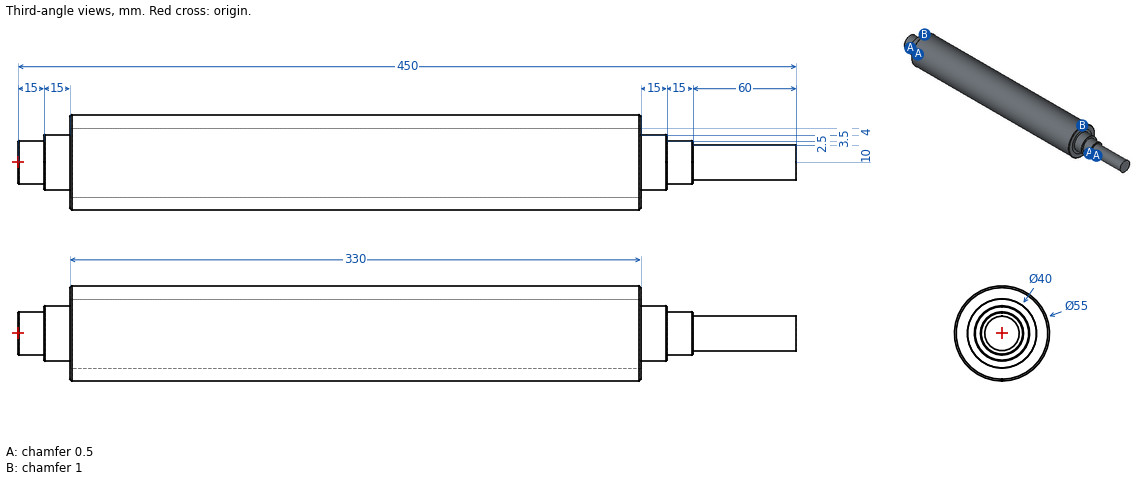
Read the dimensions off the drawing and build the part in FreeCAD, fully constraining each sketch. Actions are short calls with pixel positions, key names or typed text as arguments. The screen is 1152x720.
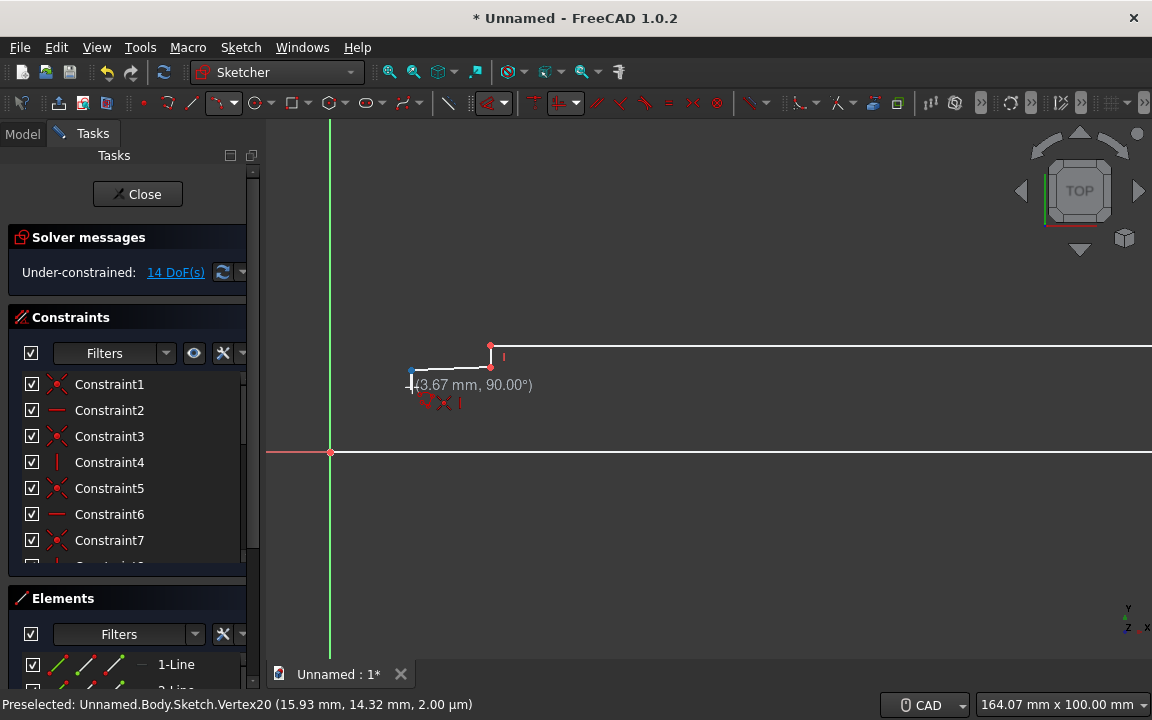
click(411, 385)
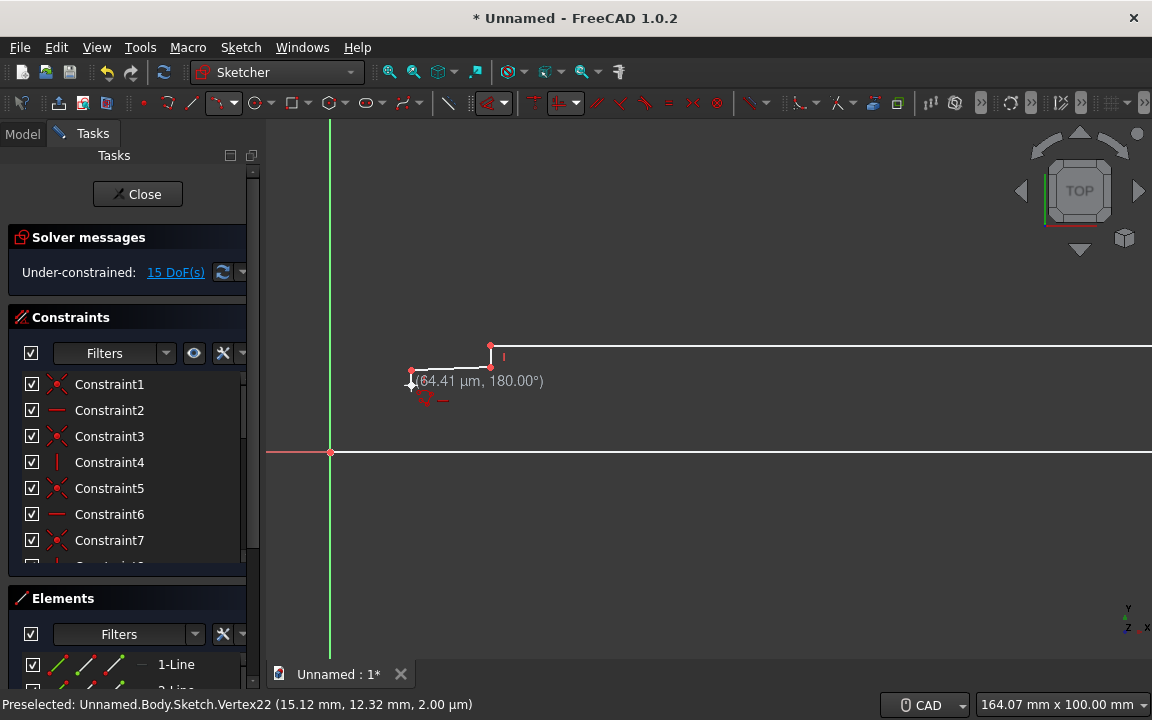
scroll(412, 387, down, 8)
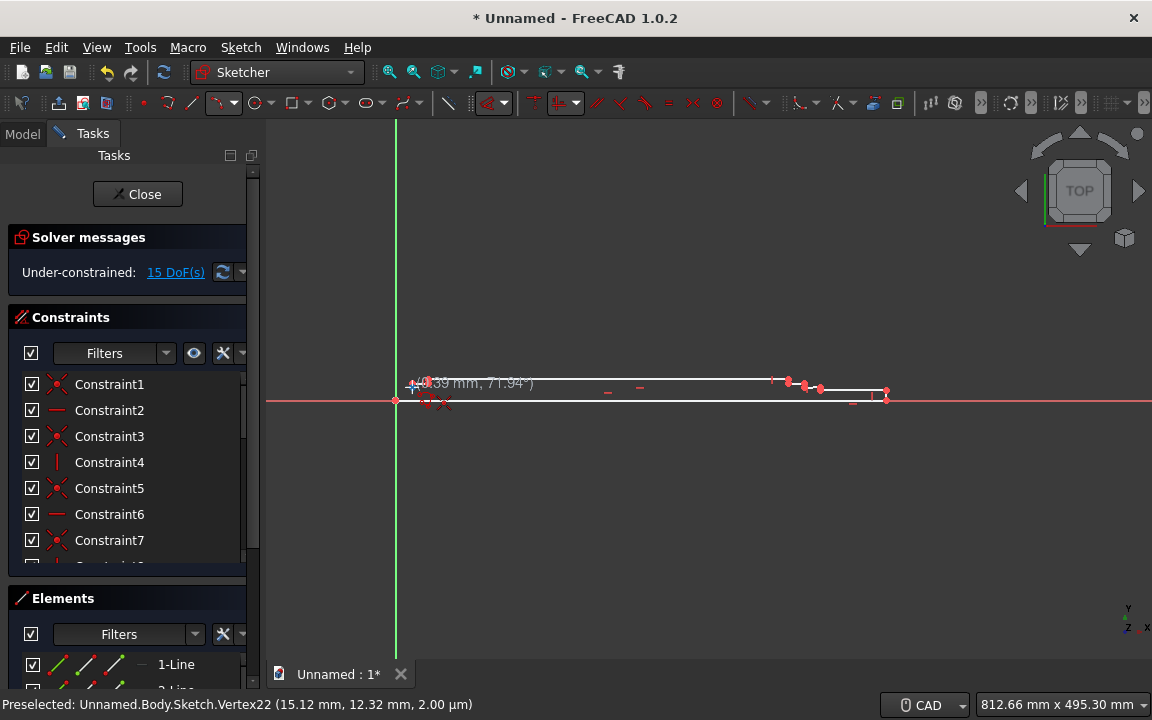
click(405, 387)
click(396, 401)
key(Escape)
key(Escape)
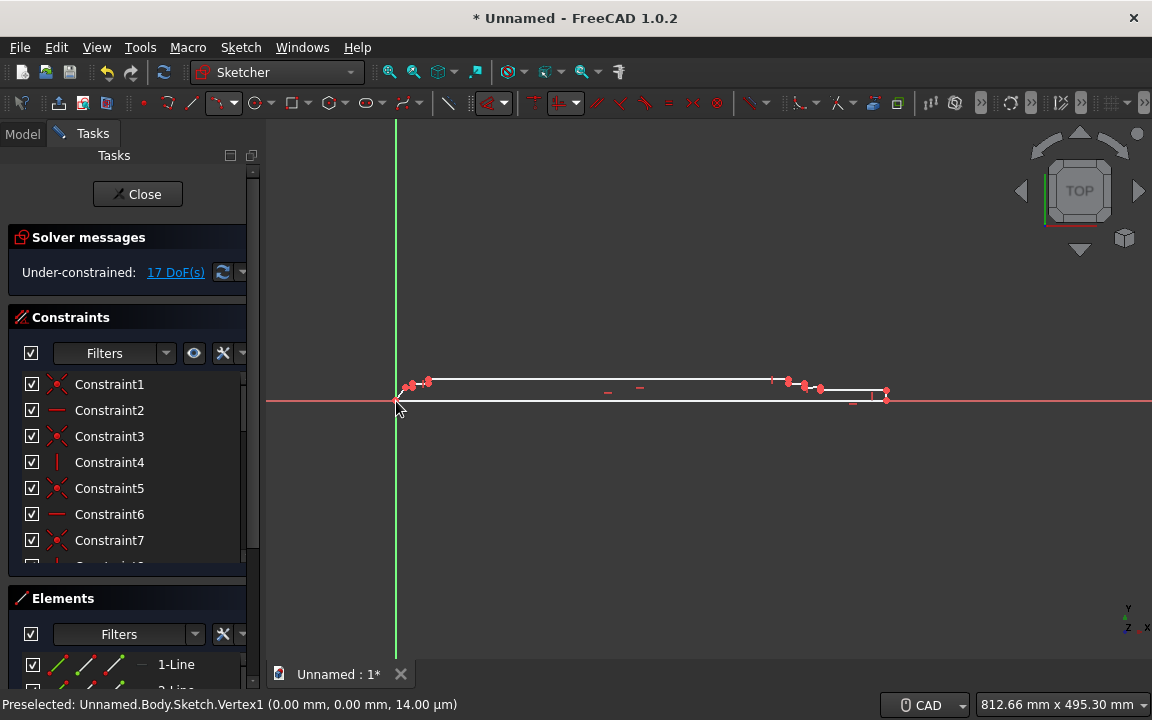
scroll(812, 388, up, 3)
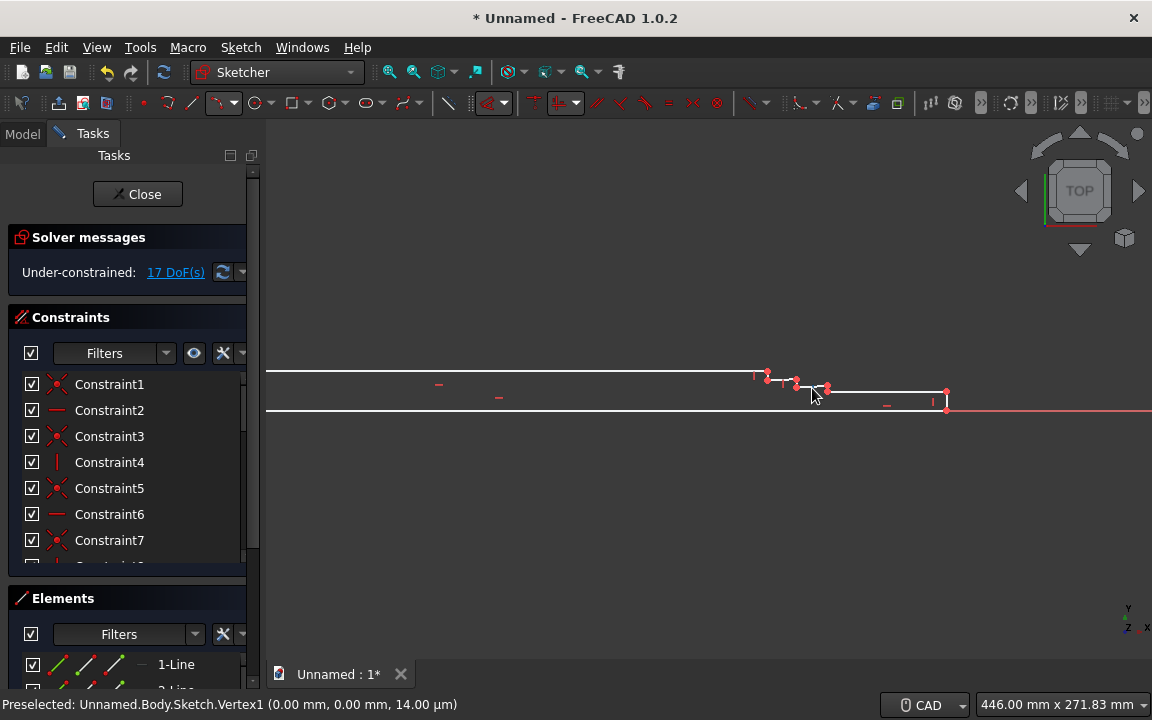
click(806, 387)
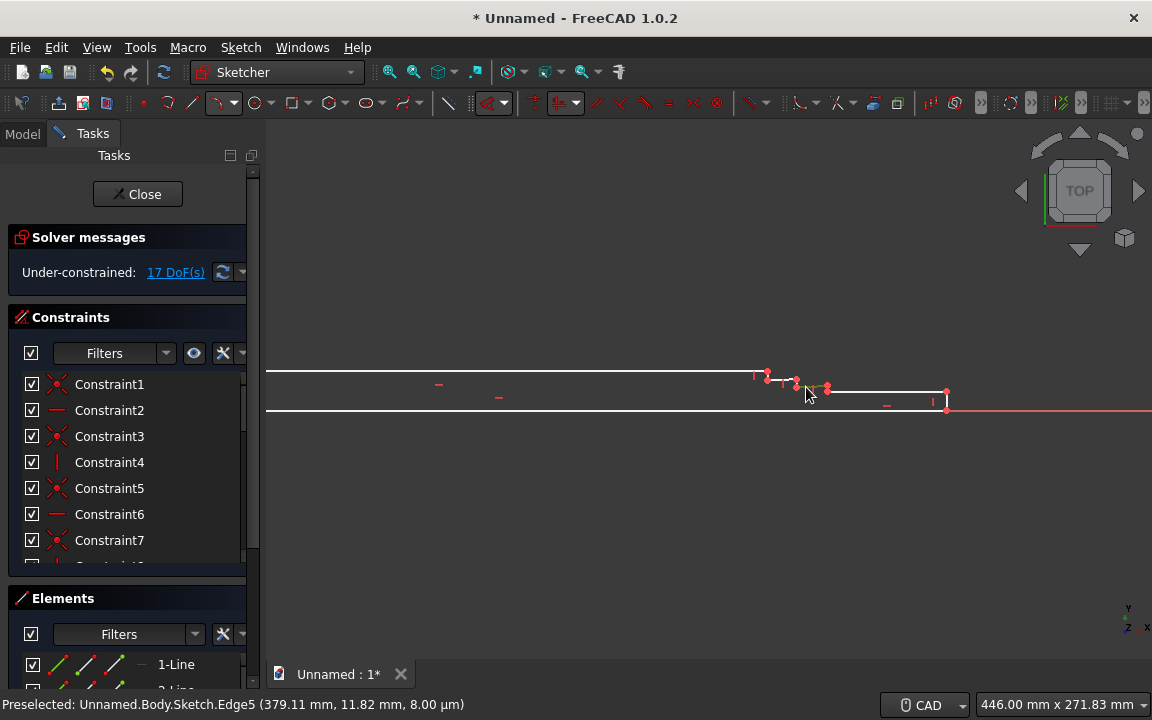
key(h)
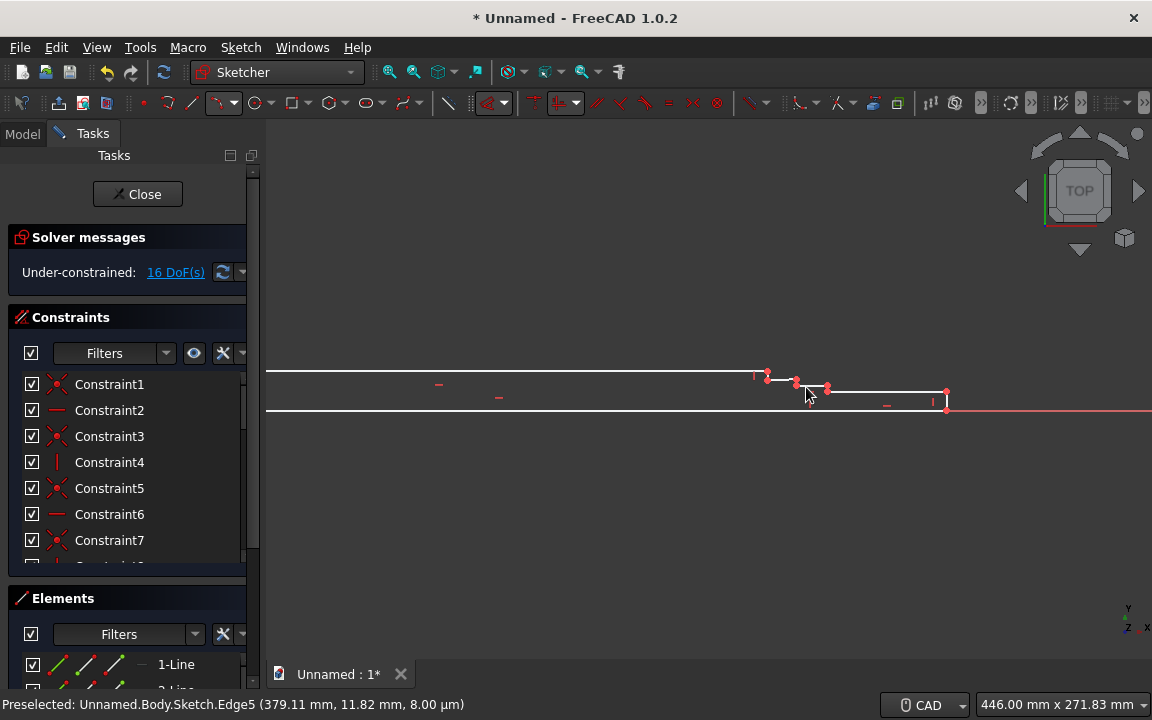
click(785, 380)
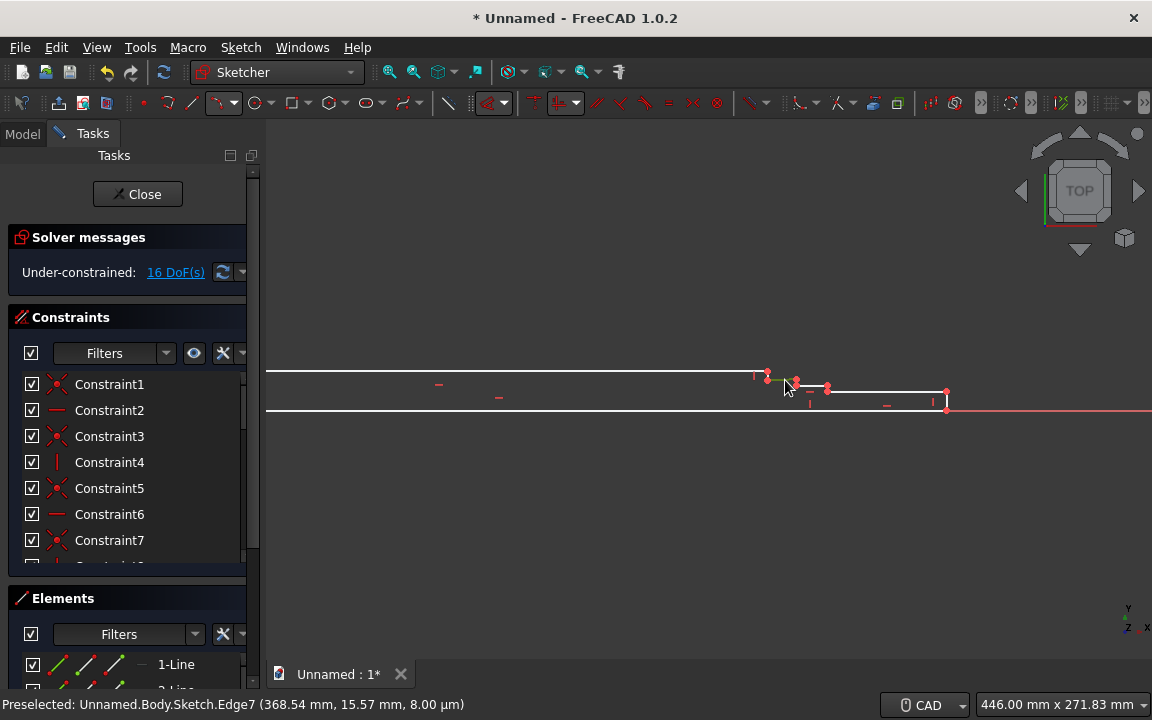
click(578, 104)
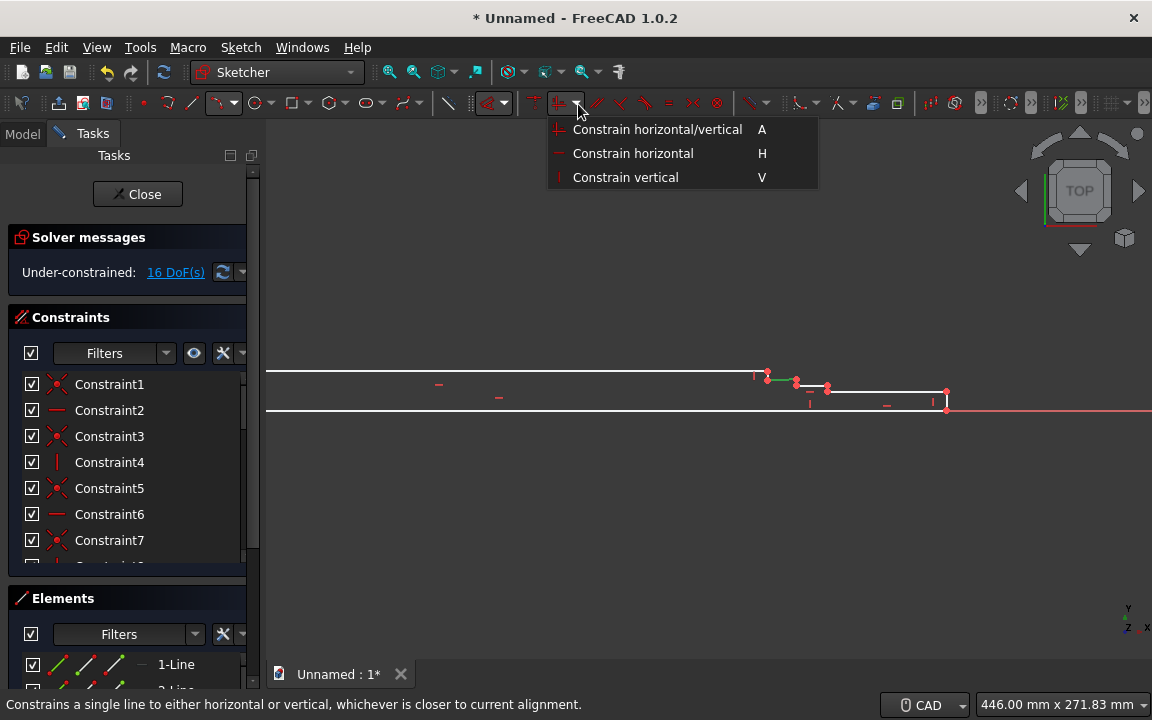
click(683, 153)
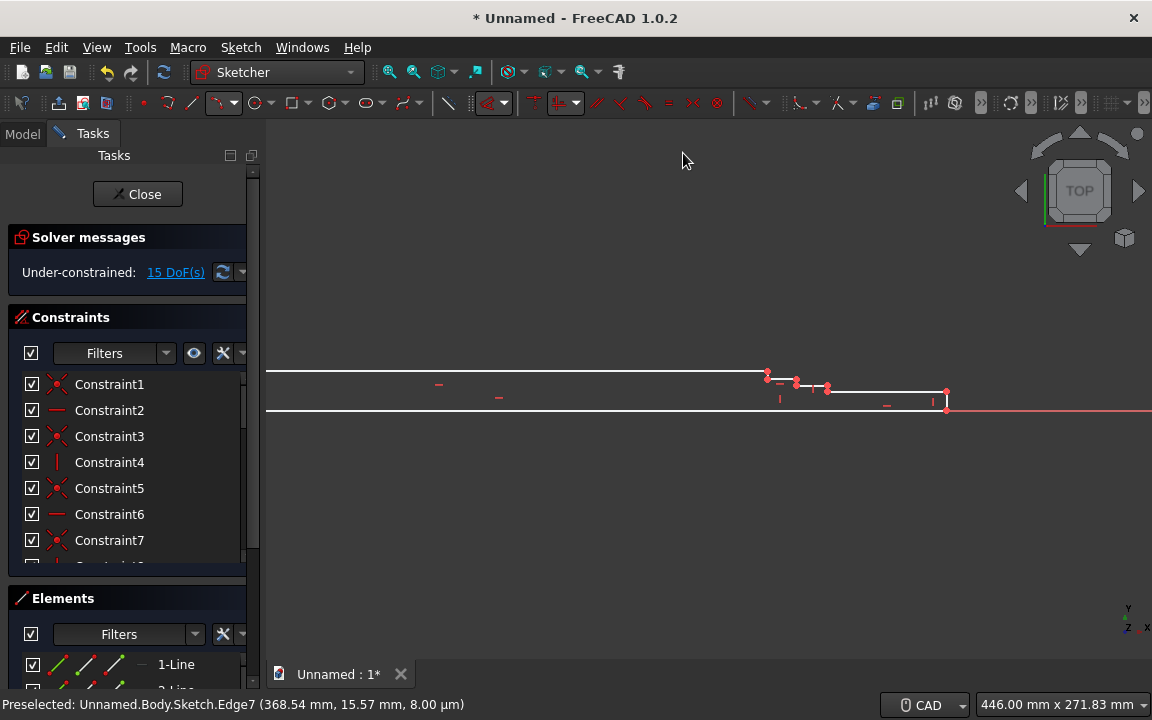
scroll(812, 387, down, 3)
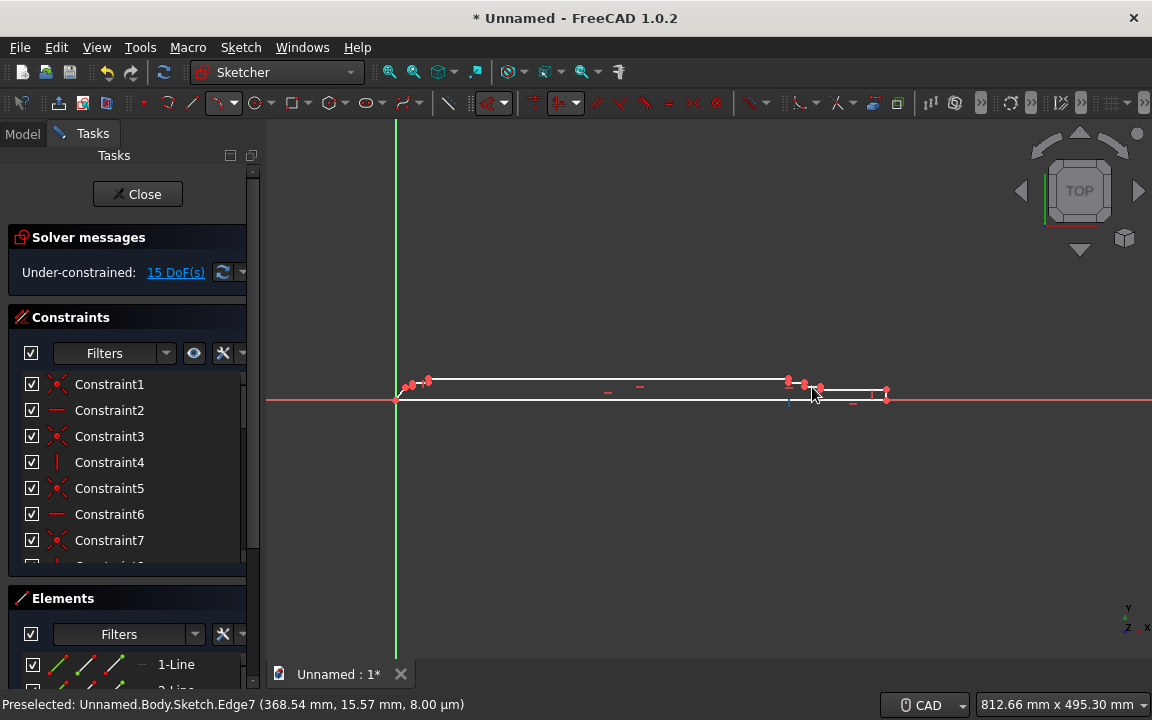
scroll(422, 383, up, 4)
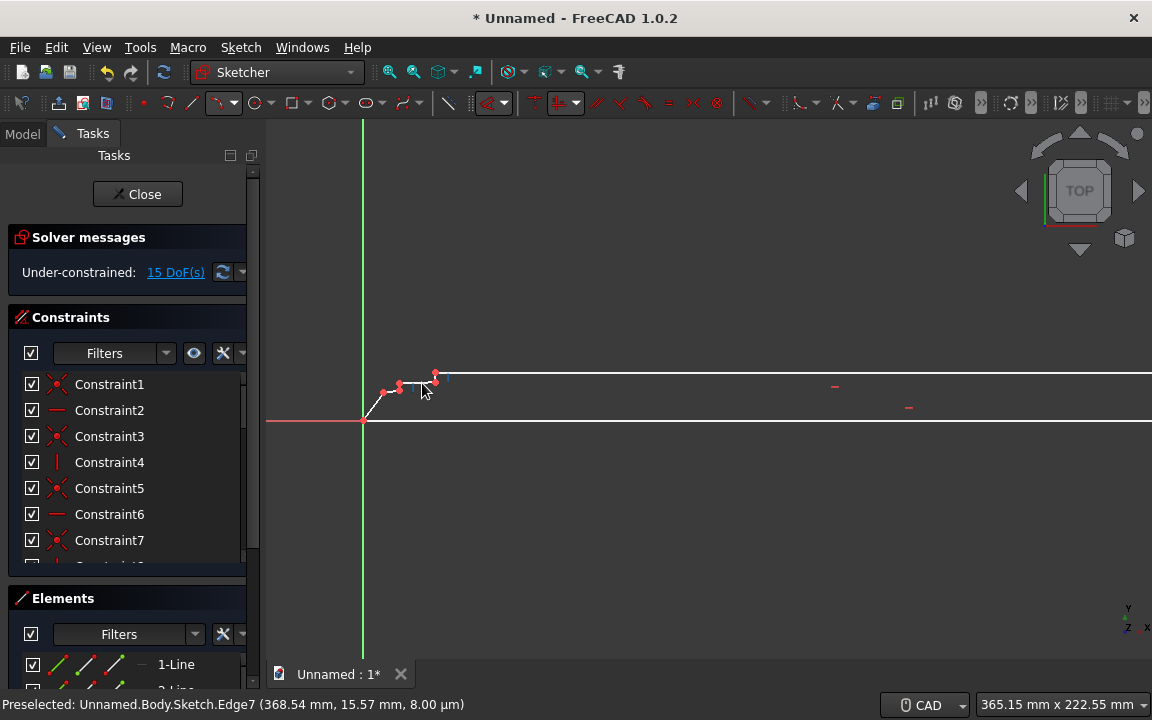
click(421, 383)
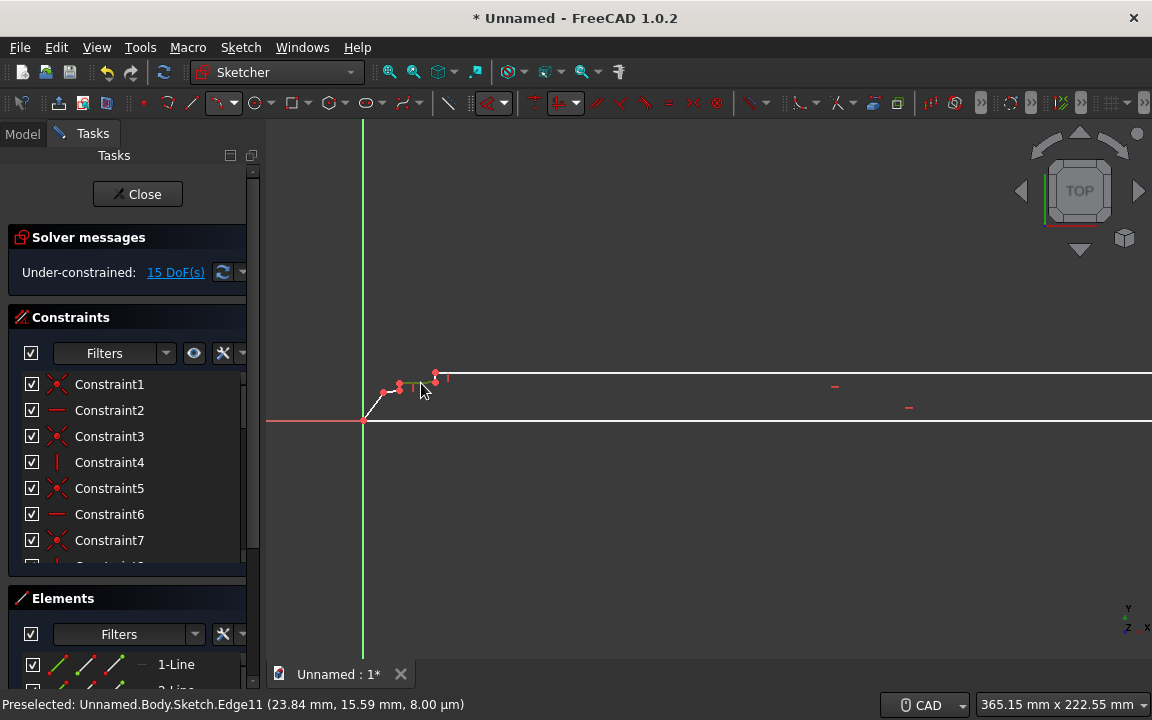
click(578, 104)